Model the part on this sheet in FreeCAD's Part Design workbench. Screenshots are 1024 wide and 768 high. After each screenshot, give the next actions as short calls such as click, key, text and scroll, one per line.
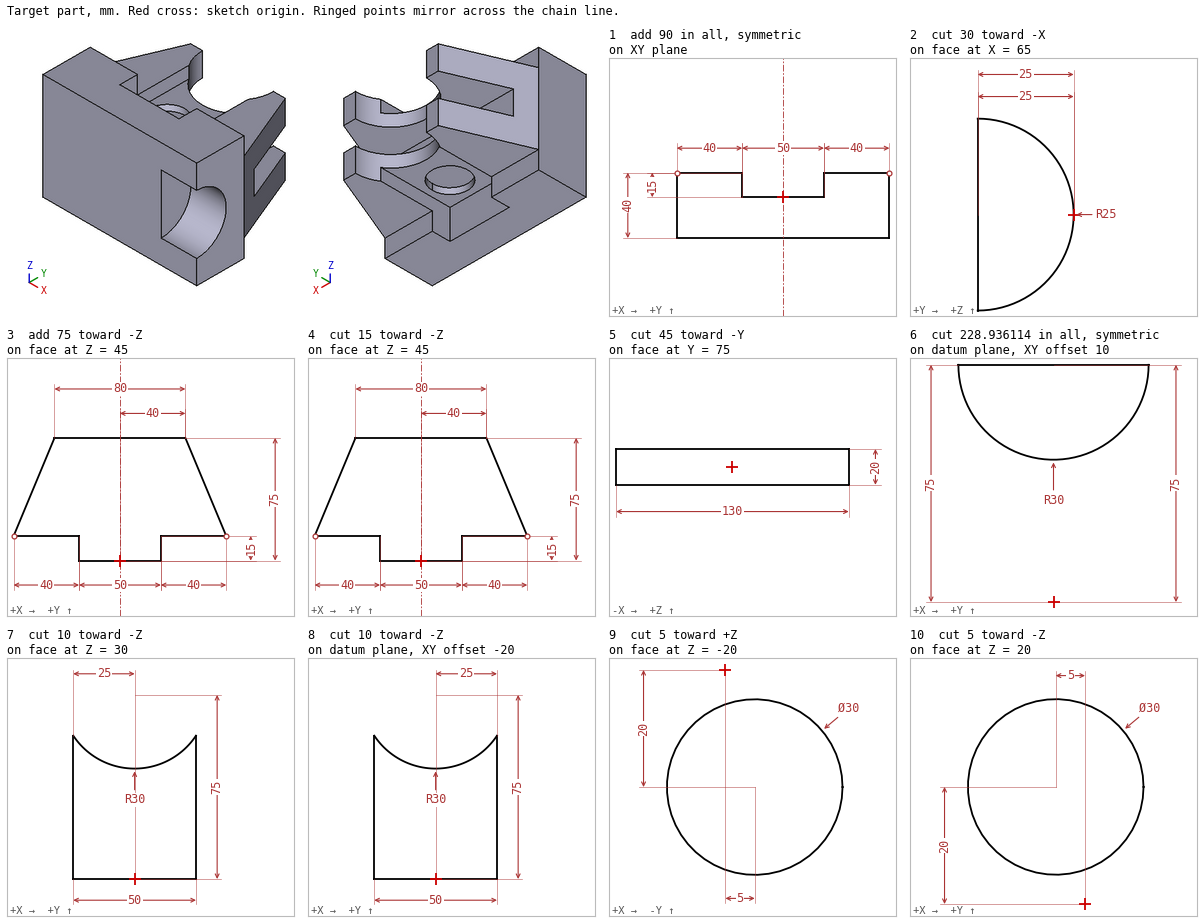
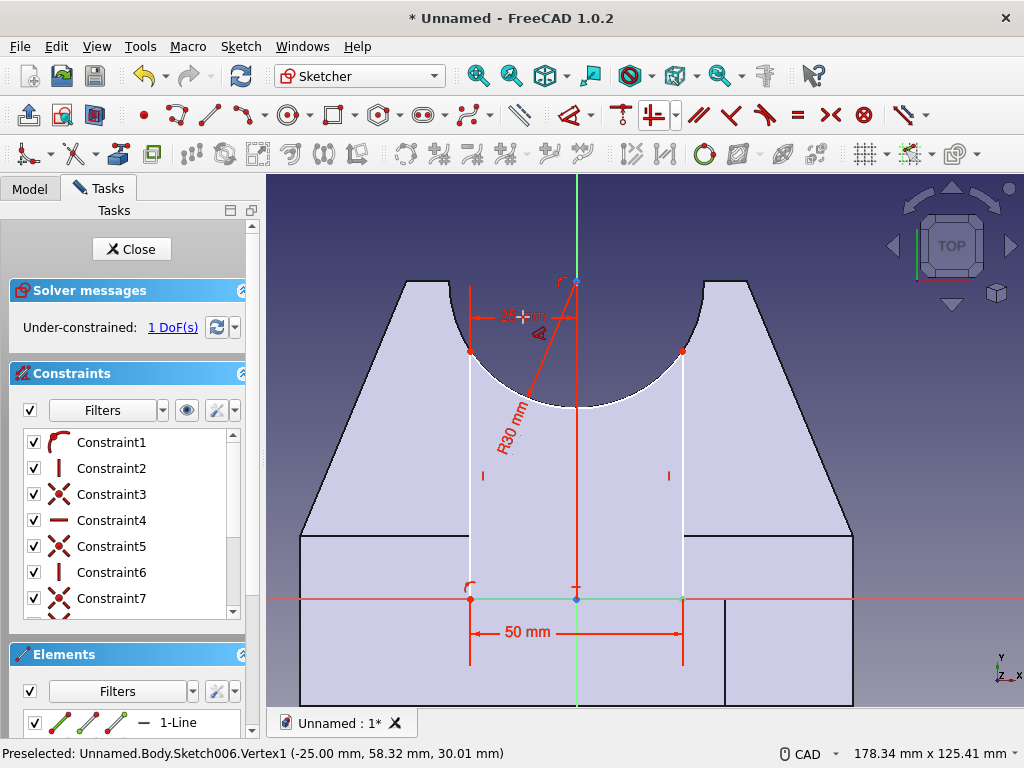
click(577, 281)
click(611, 440)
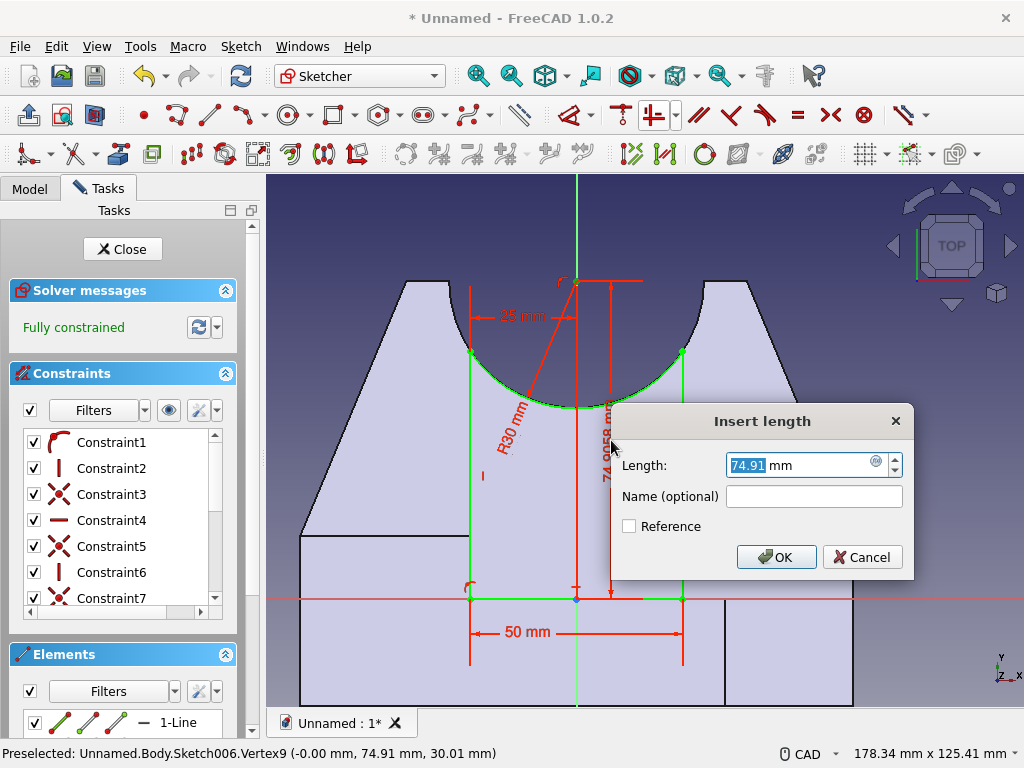
text(75)
key(Return)
key(Escape)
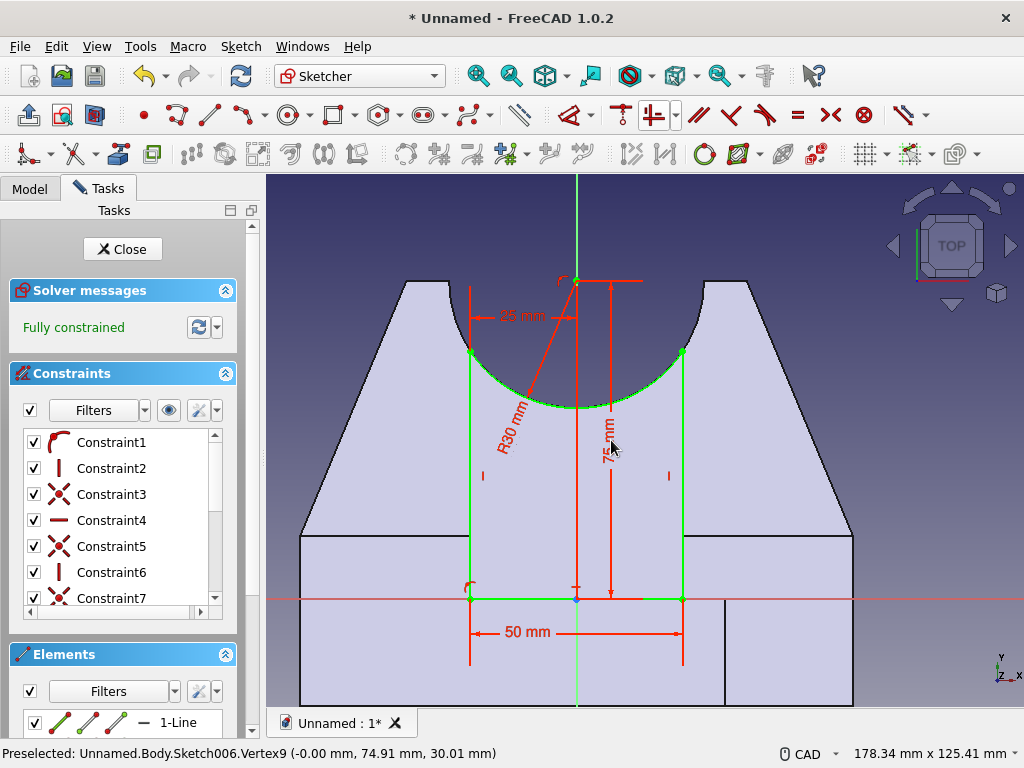
click(123, 249)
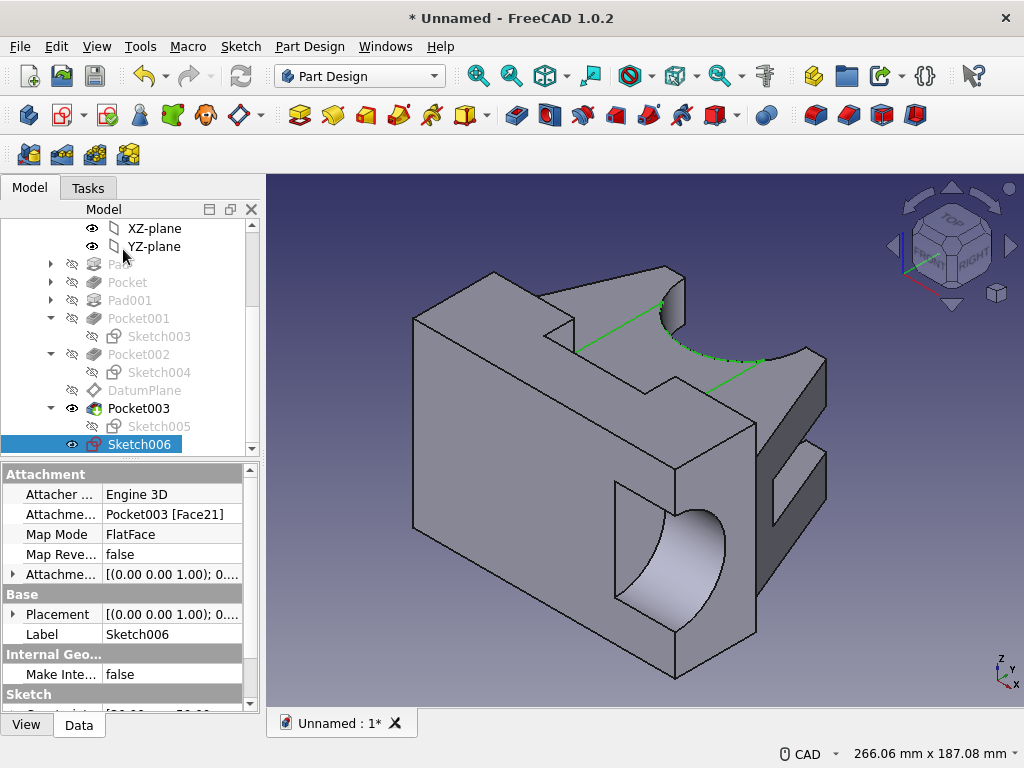
click(517, 116)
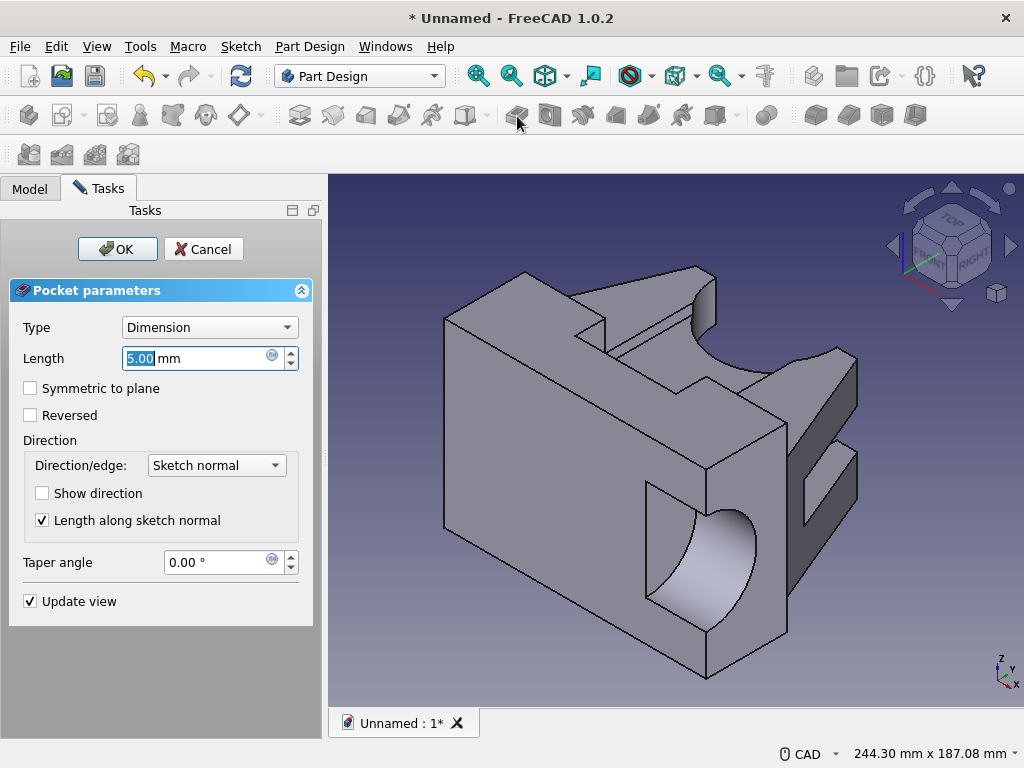
text(10)
key(Tab)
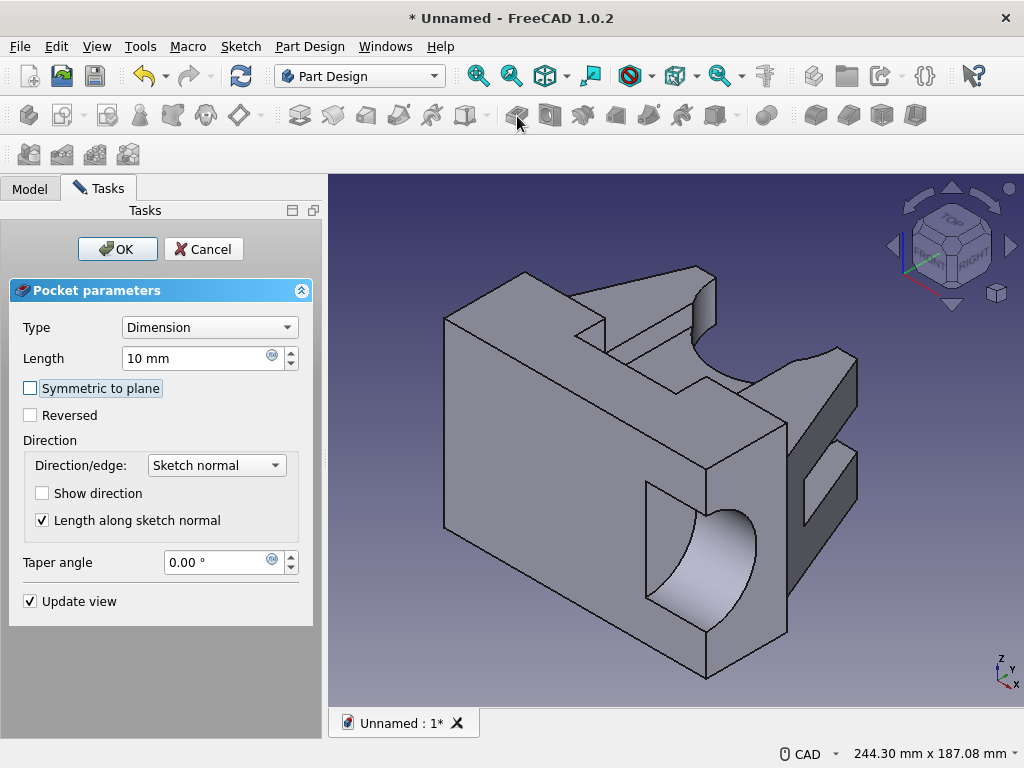
click(118, 249)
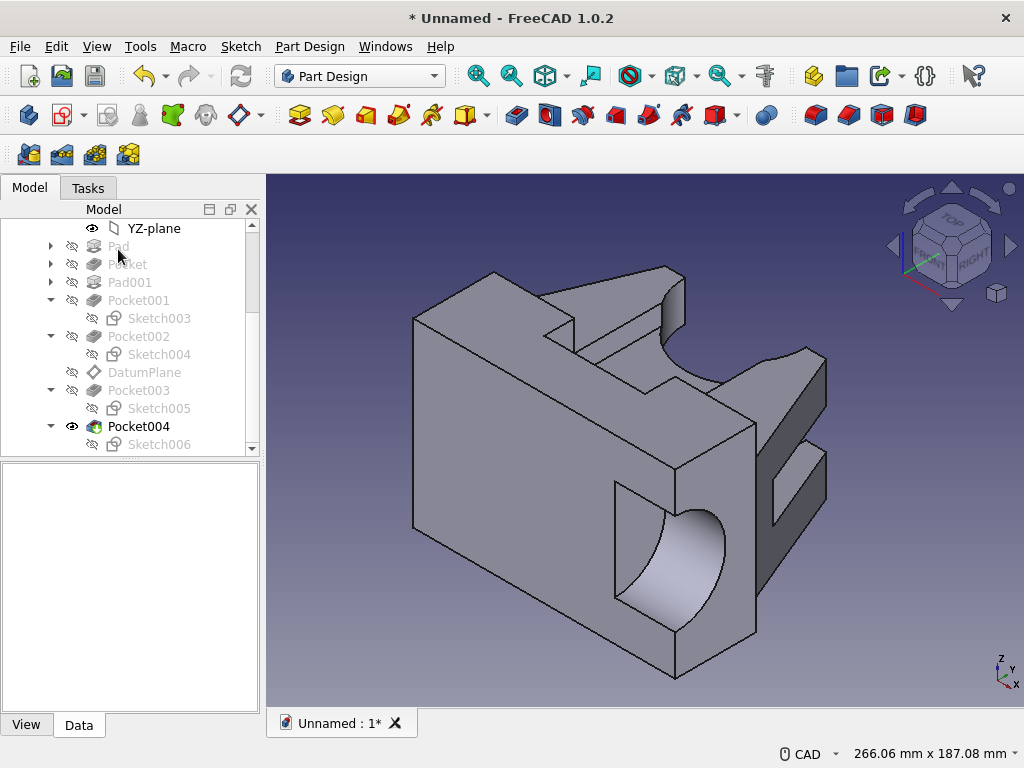
scroll(161, 332, down, 3)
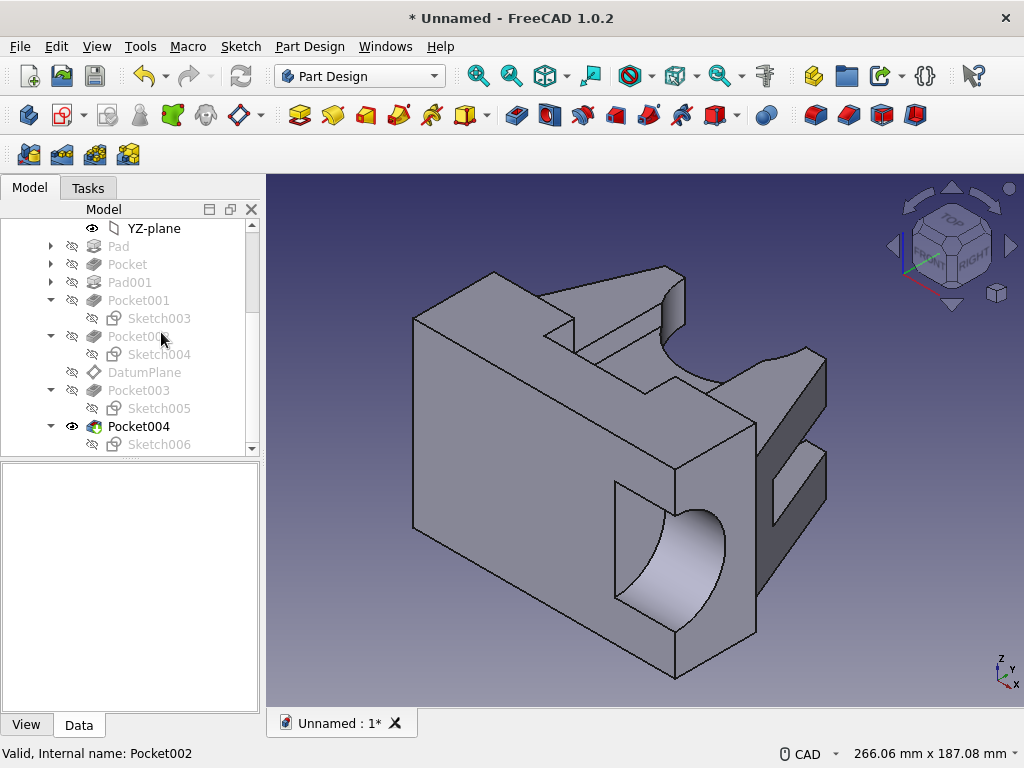
scroll(161, 332, up, 15)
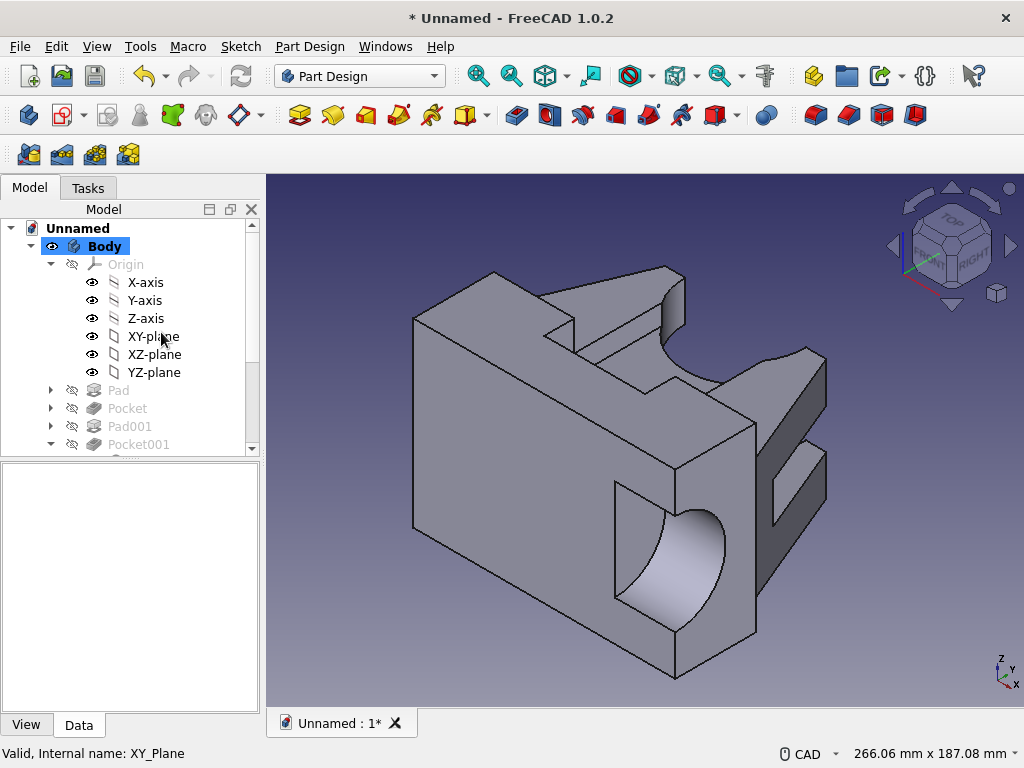
click(137, 336)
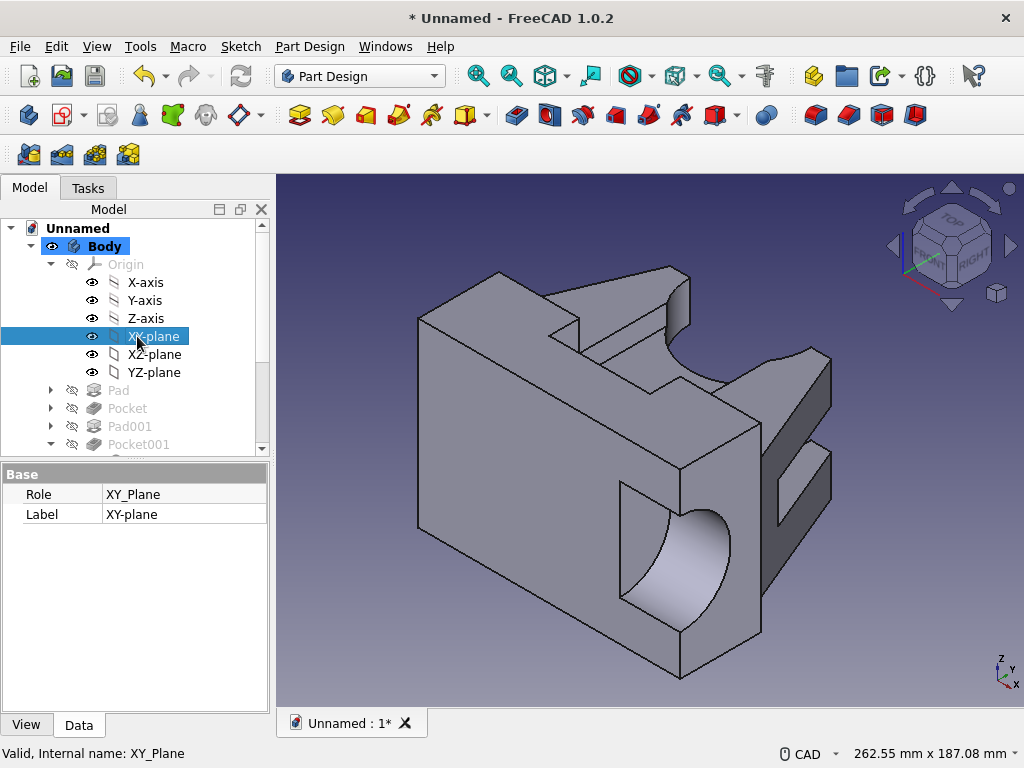
click(238, 116)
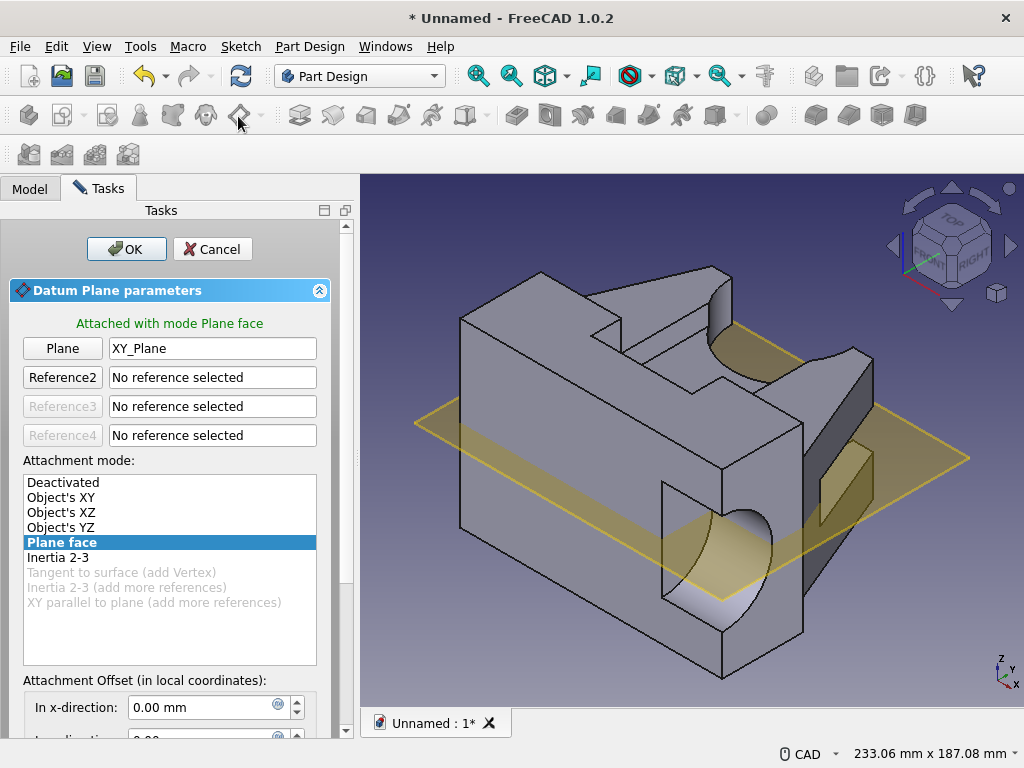
scroll(346, 479, down, 2)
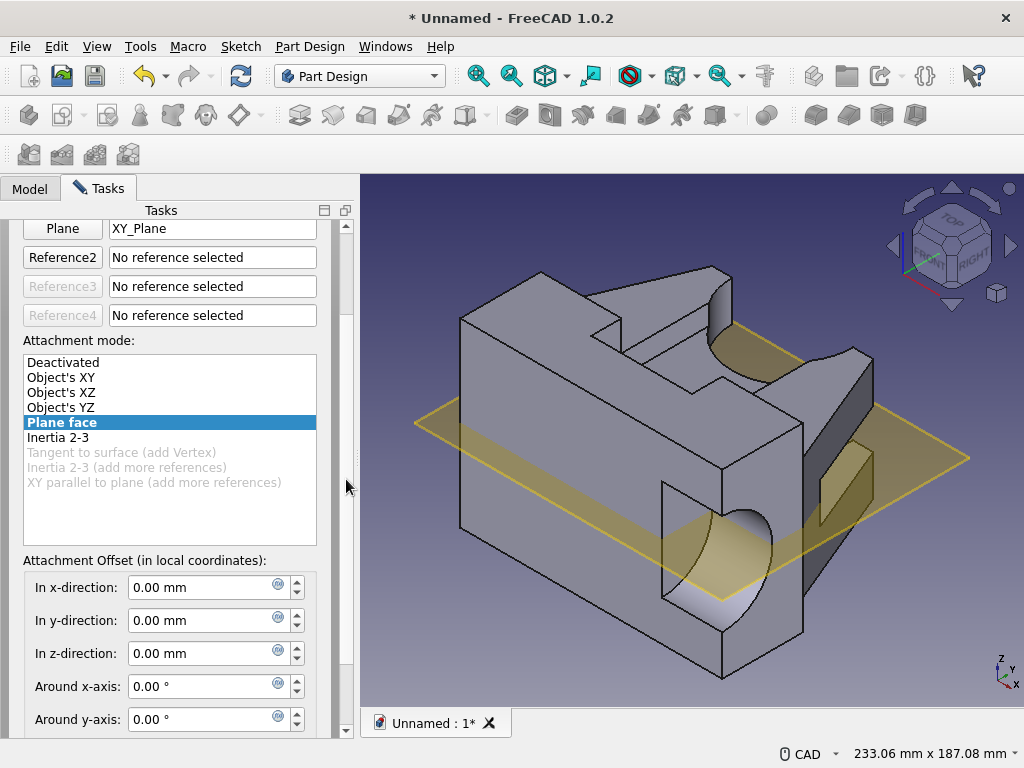
triple_click(210, 654)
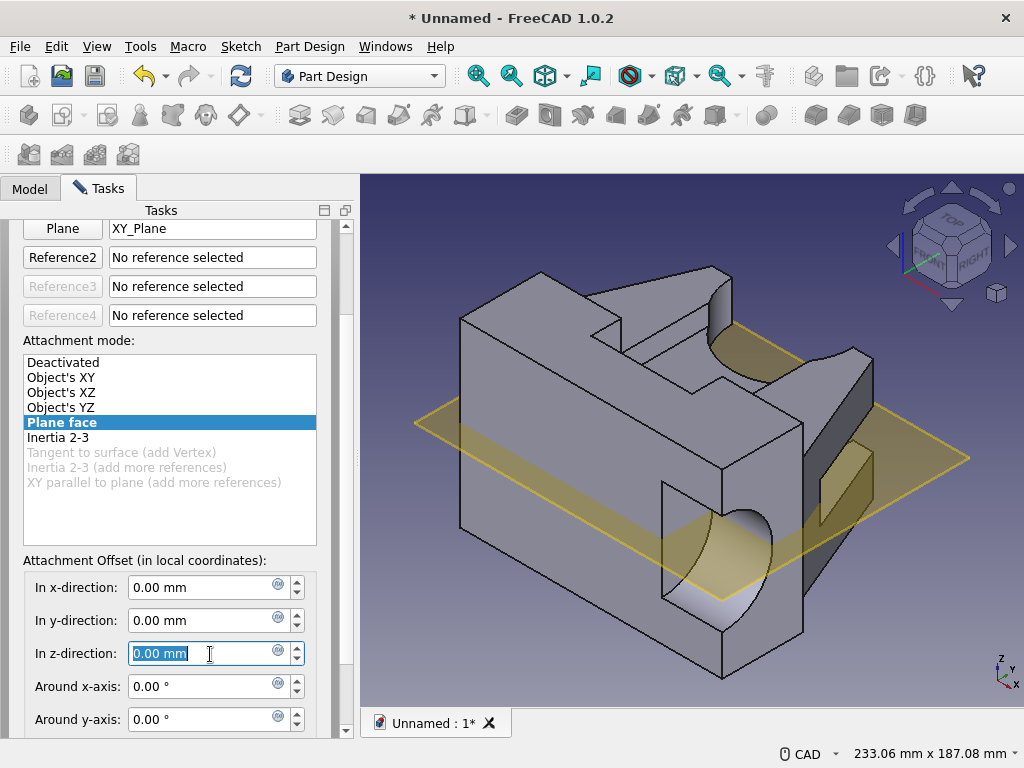
text(-20)
key(Tab)